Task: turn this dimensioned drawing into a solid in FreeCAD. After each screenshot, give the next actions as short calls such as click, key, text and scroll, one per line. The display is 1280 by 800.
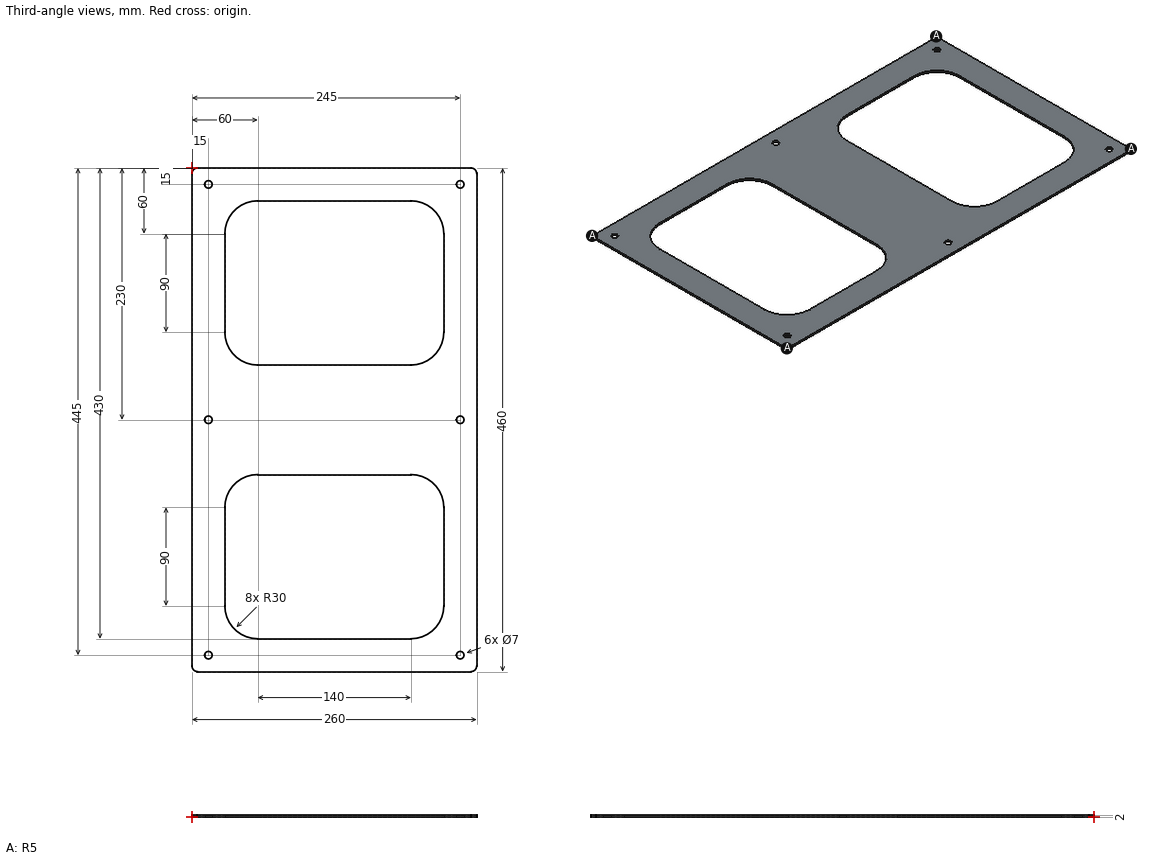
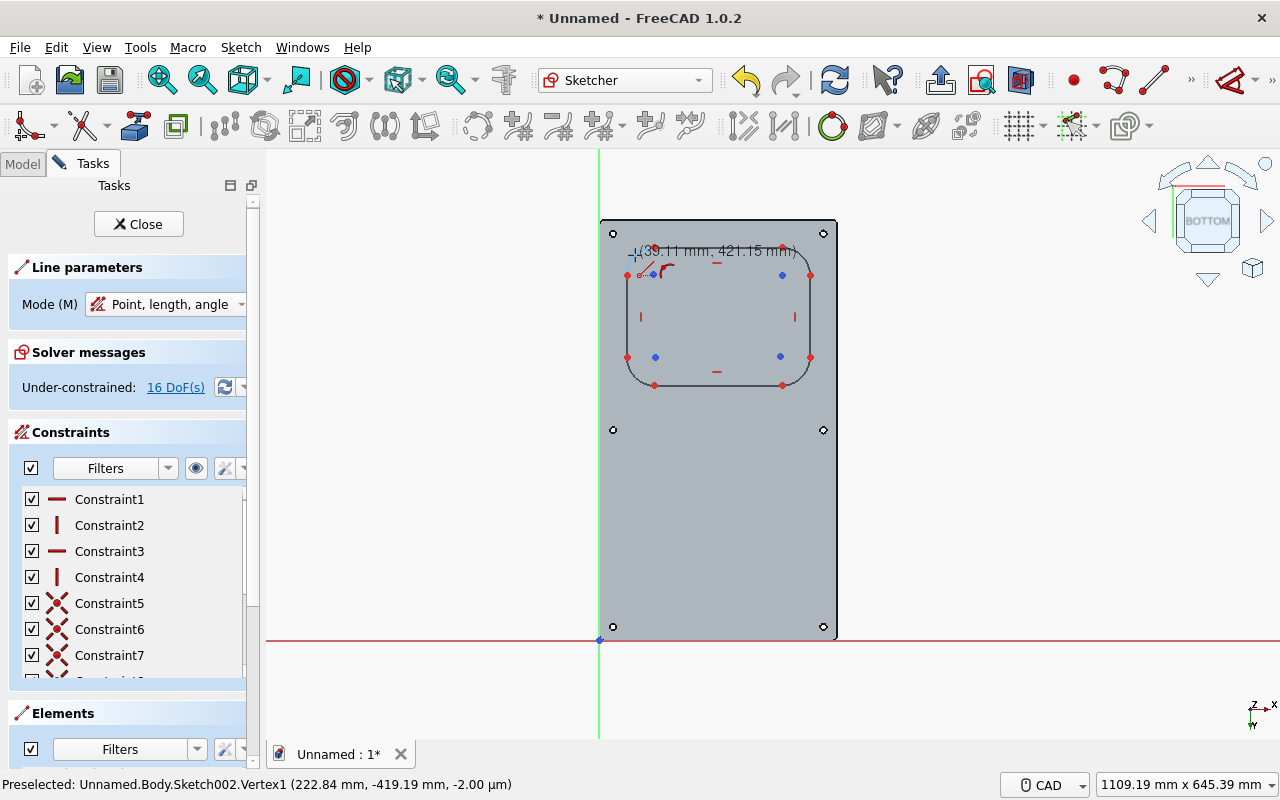
click(782, 476)
click(654, 476)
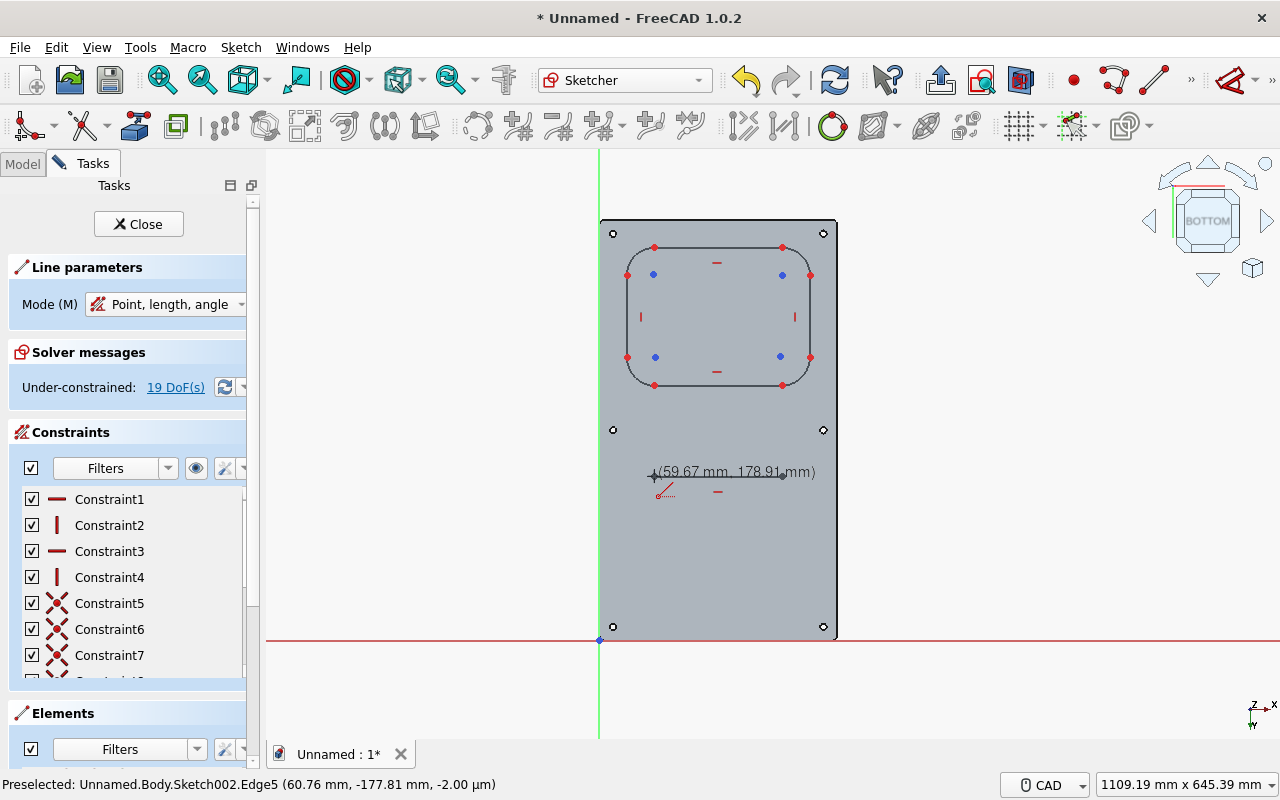
click(627, 503)
click(627, 586)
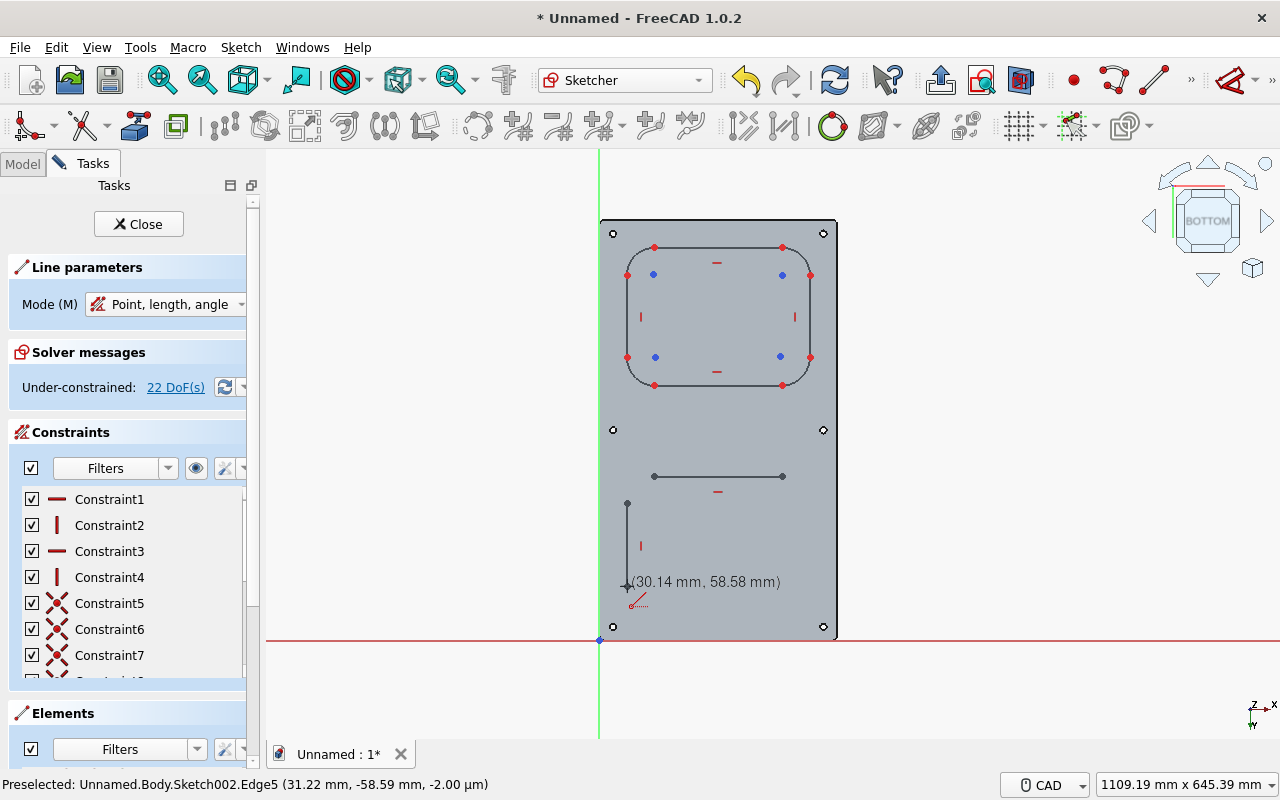
click(654, 613)
click(782, 613)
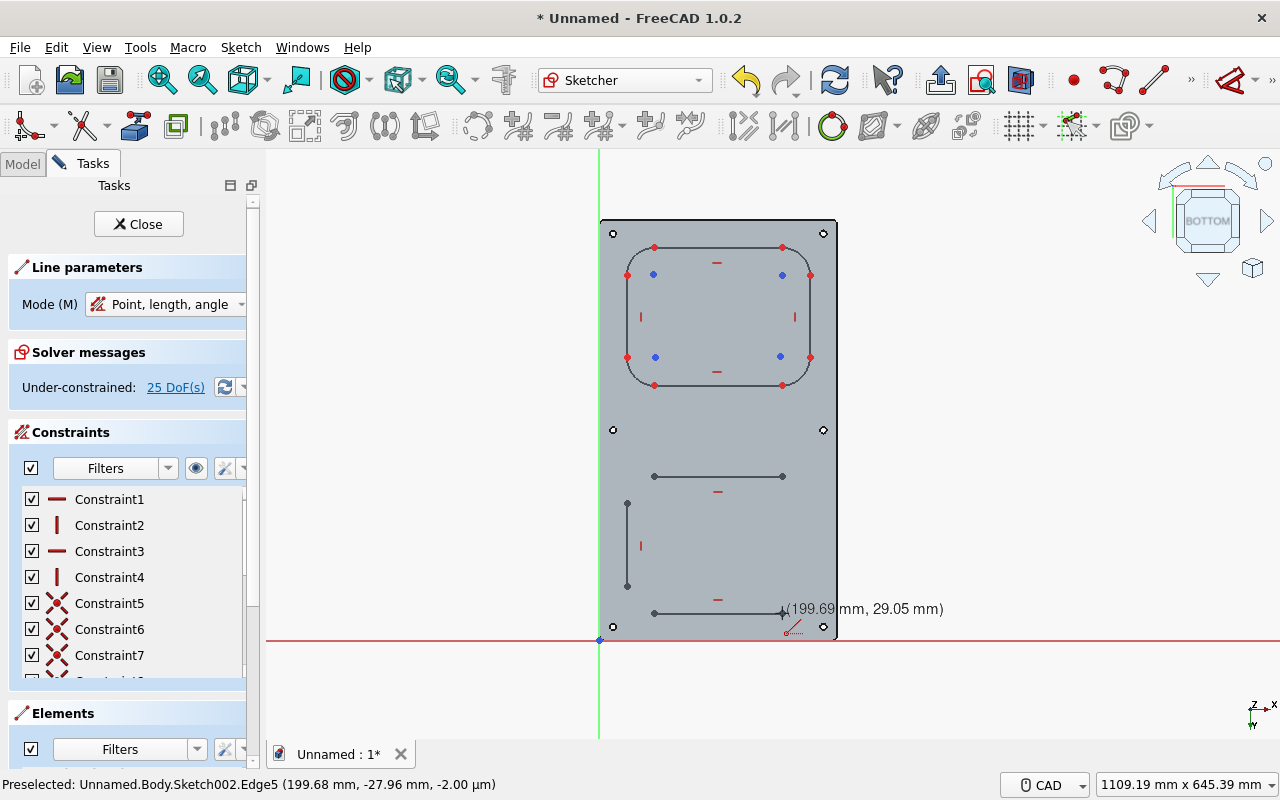
click(810, 586)
click(810, 503)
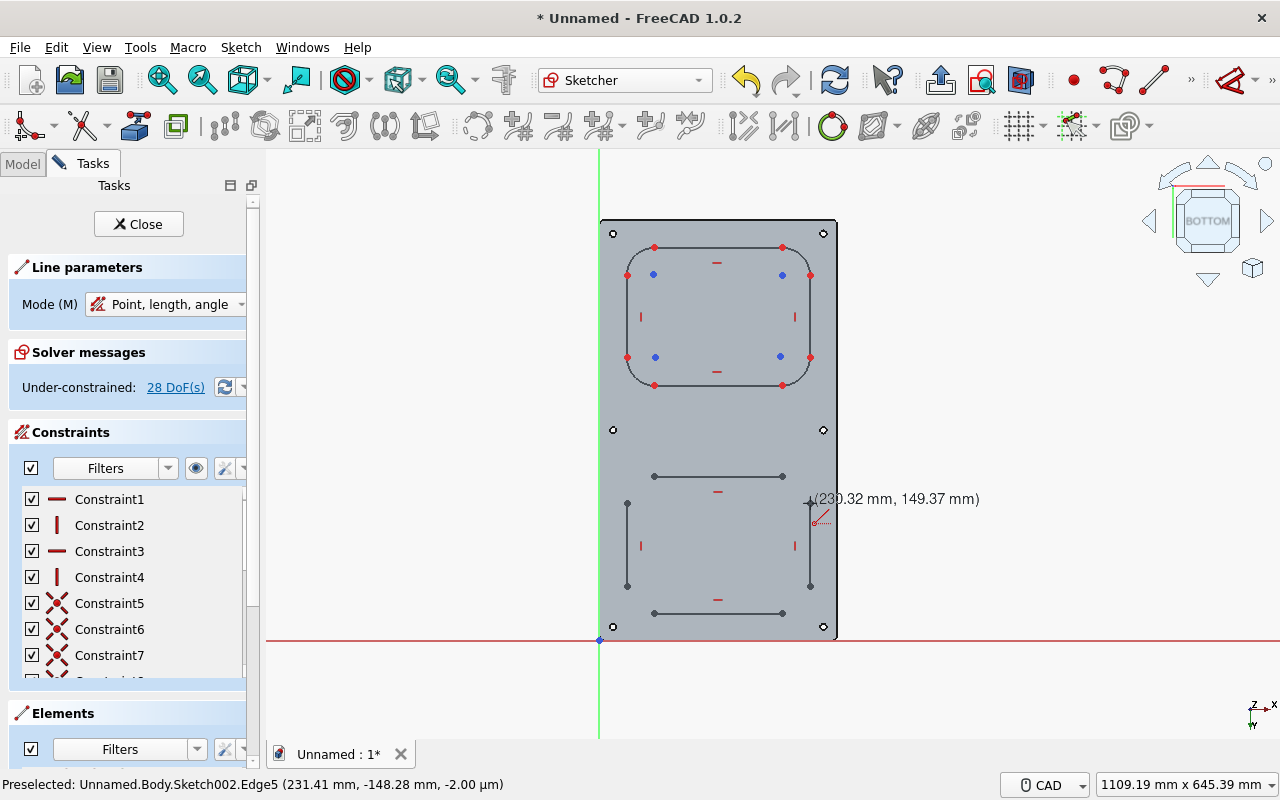
key(g)
key(3)
key(a)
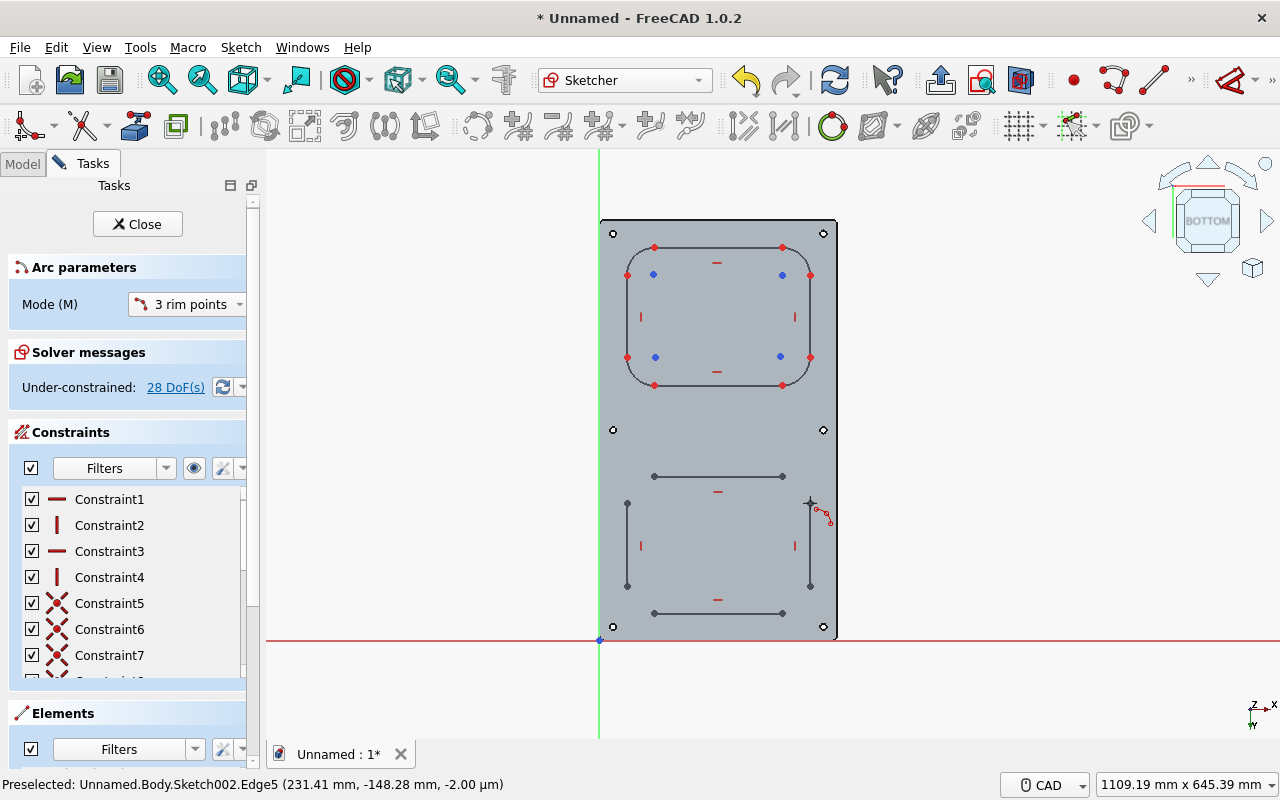
click(654, 477)
click(627, 504)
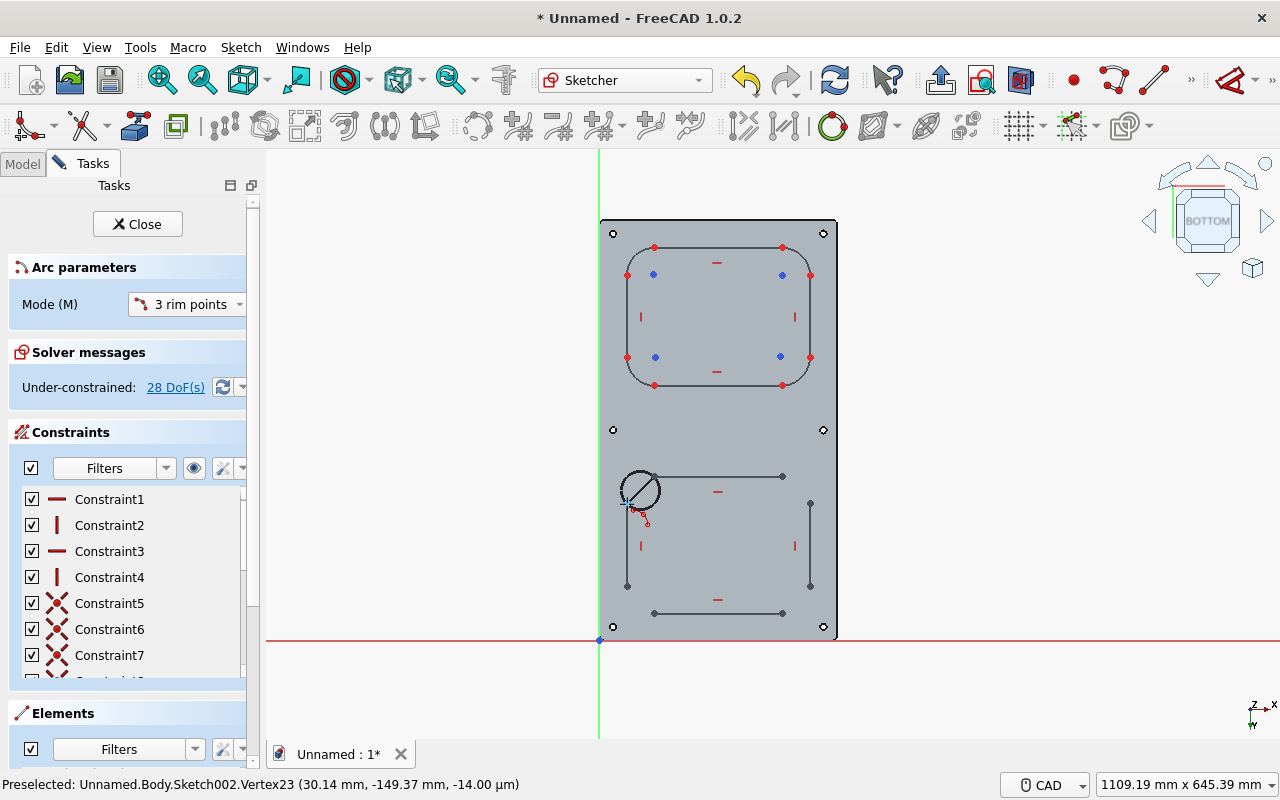
scroll(635, 484, up, 4)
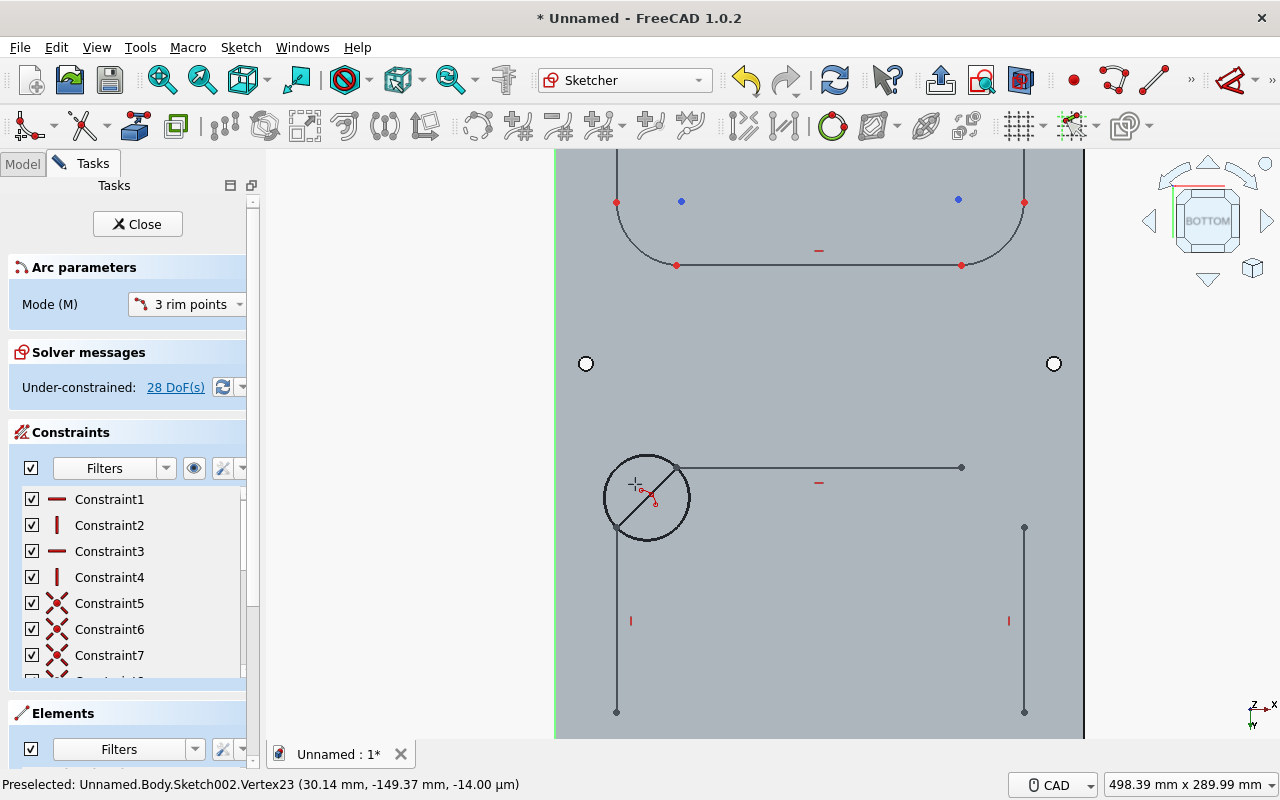
click(634, 483)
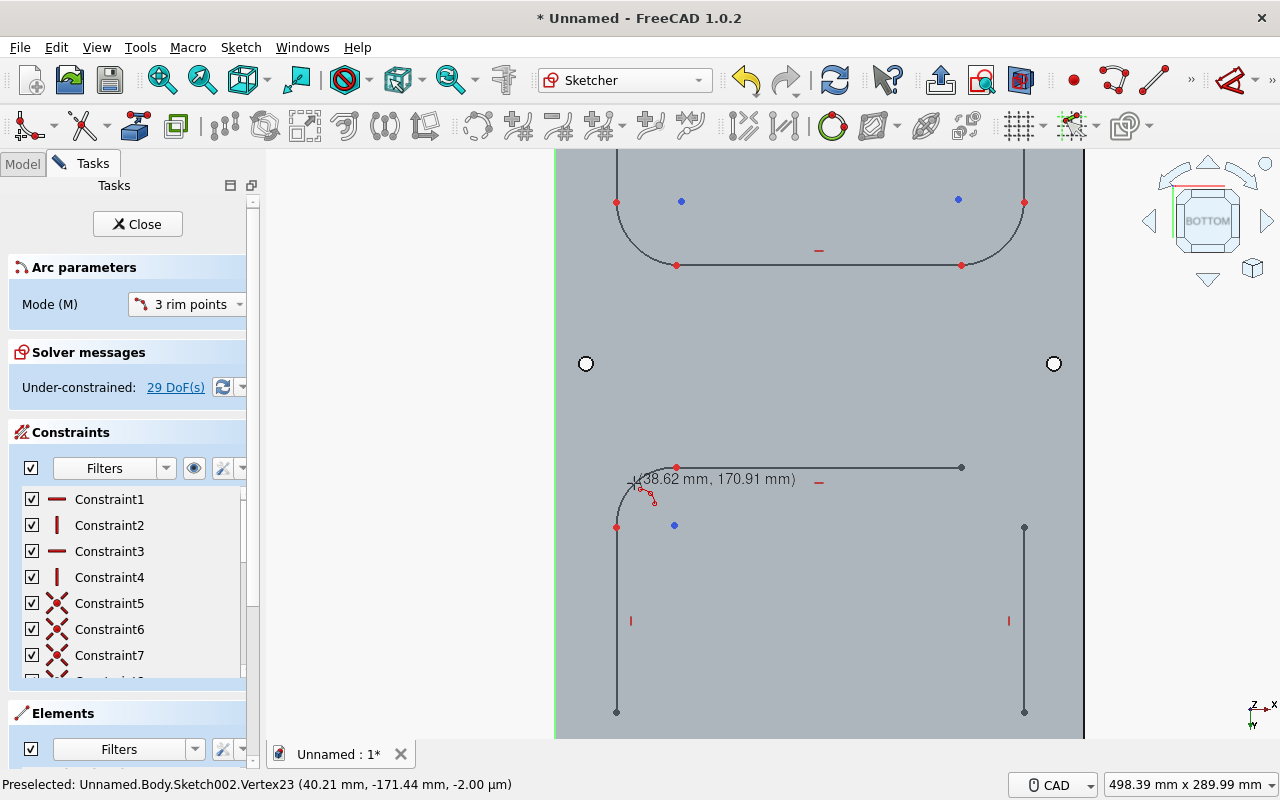
click(617, 713)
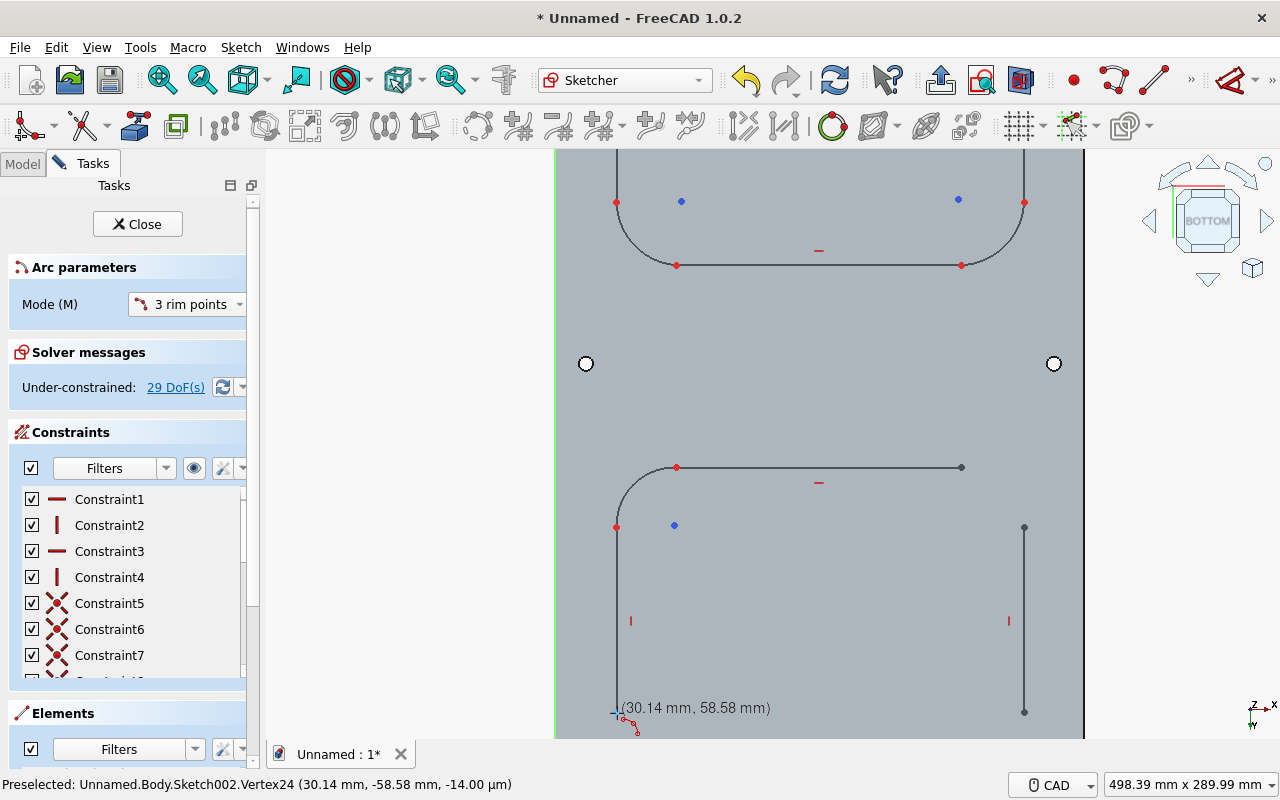
scroll(635, 485, down, 4)